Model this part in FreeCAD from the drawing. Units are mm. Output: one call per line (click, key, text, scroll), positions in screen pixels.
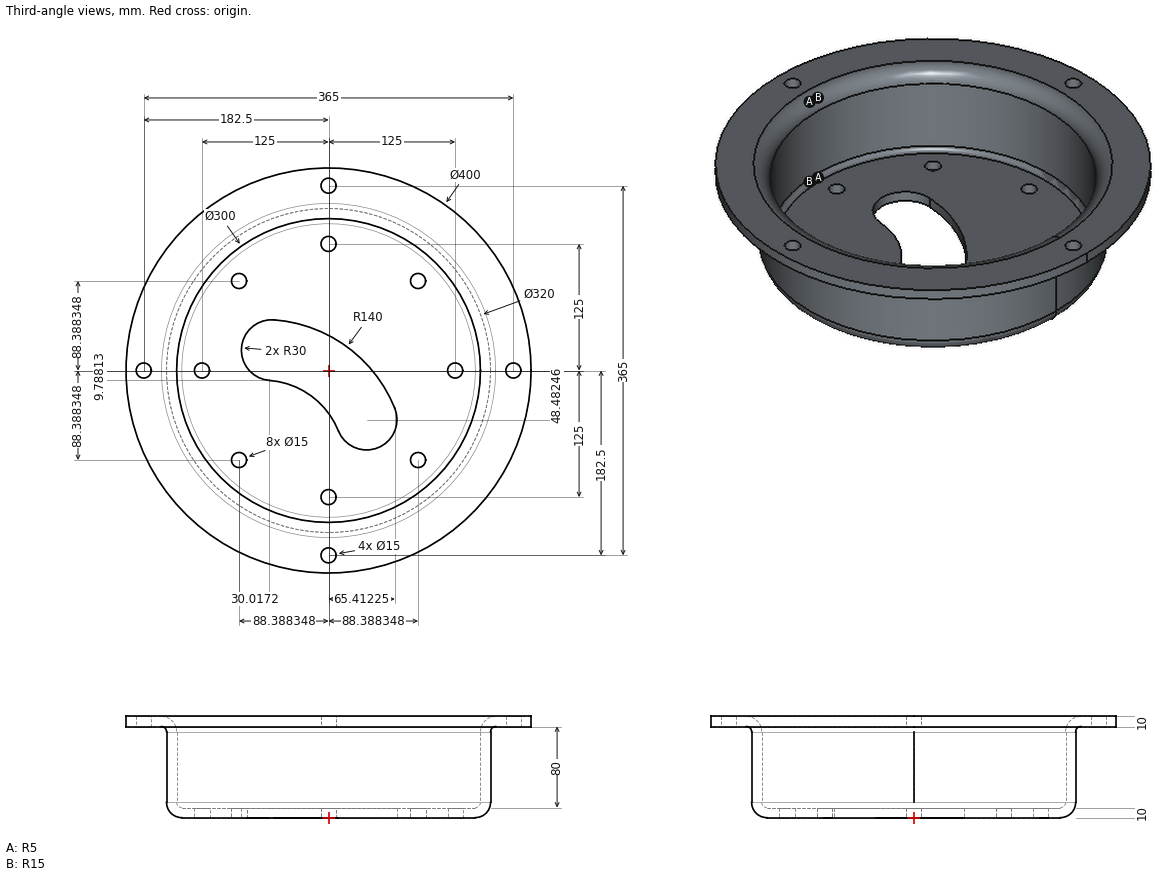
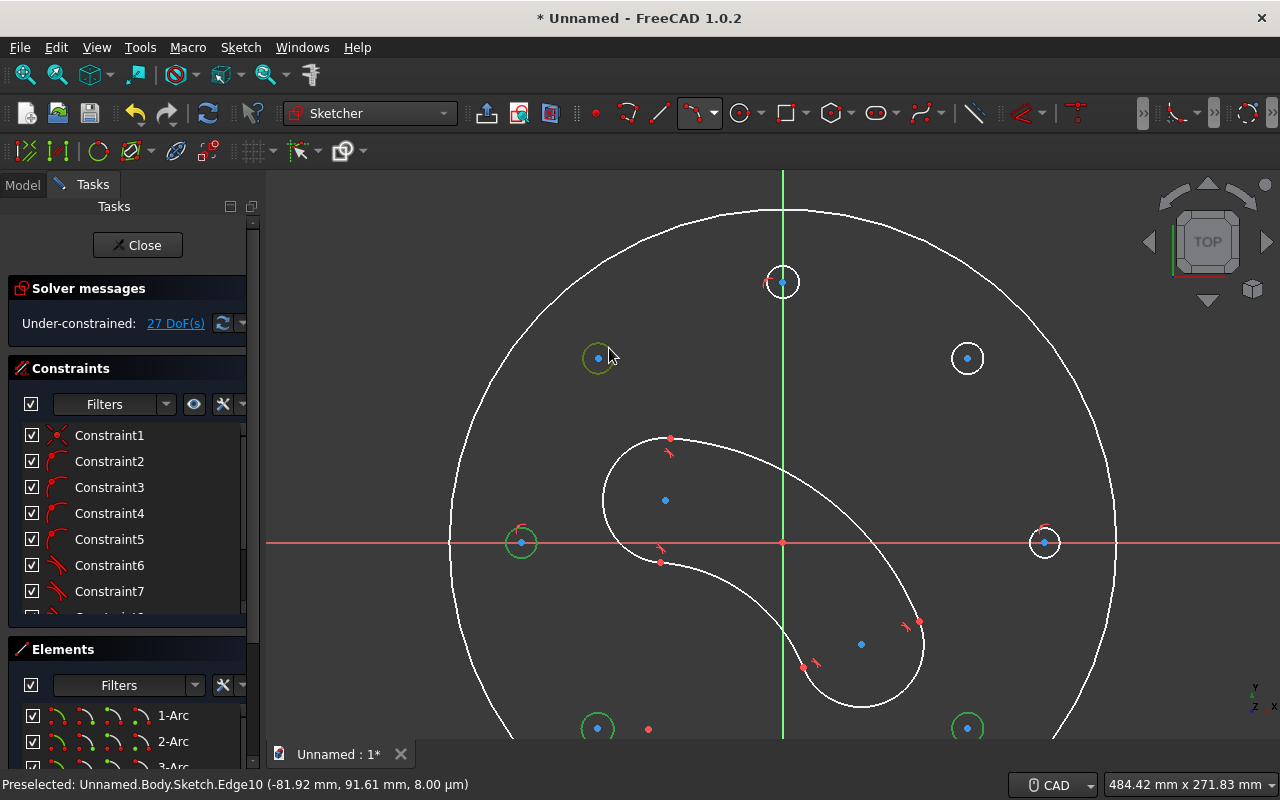
scroll(1055, 532, up, 2)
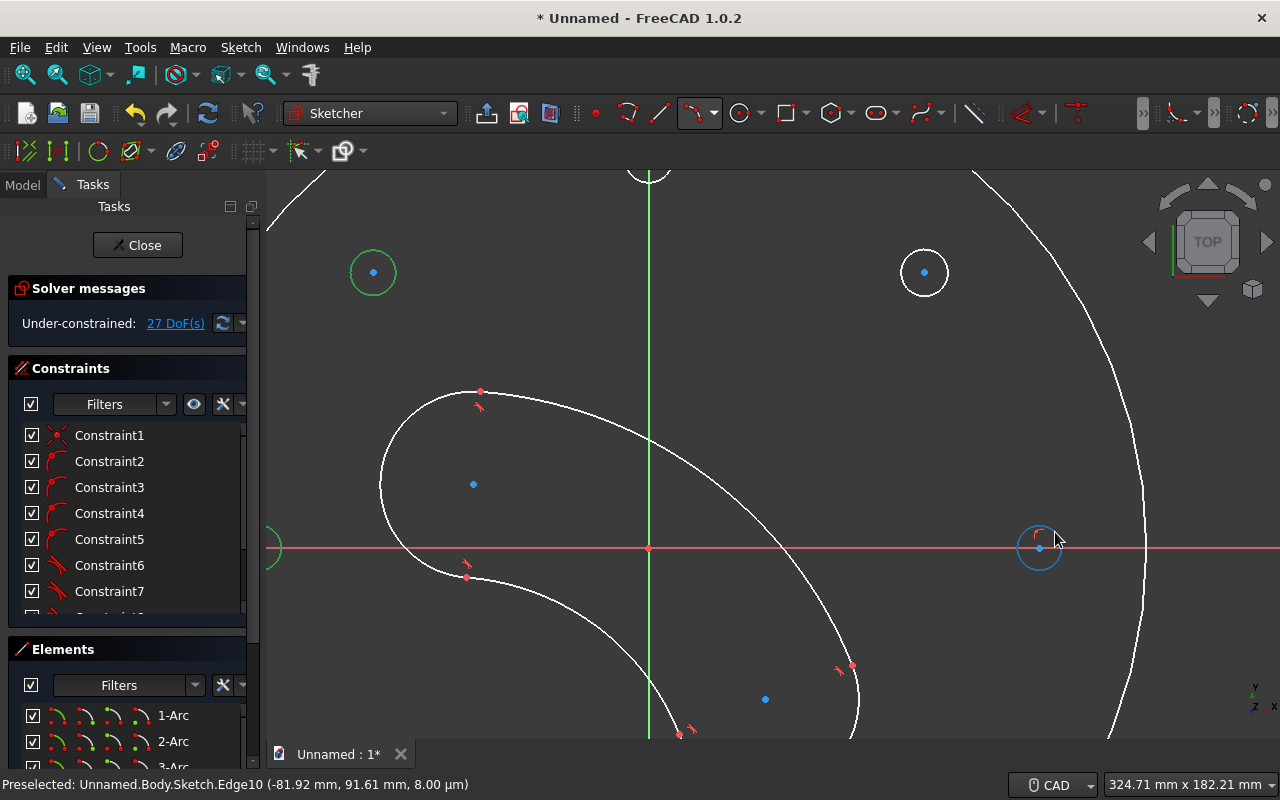
click(1055, 532)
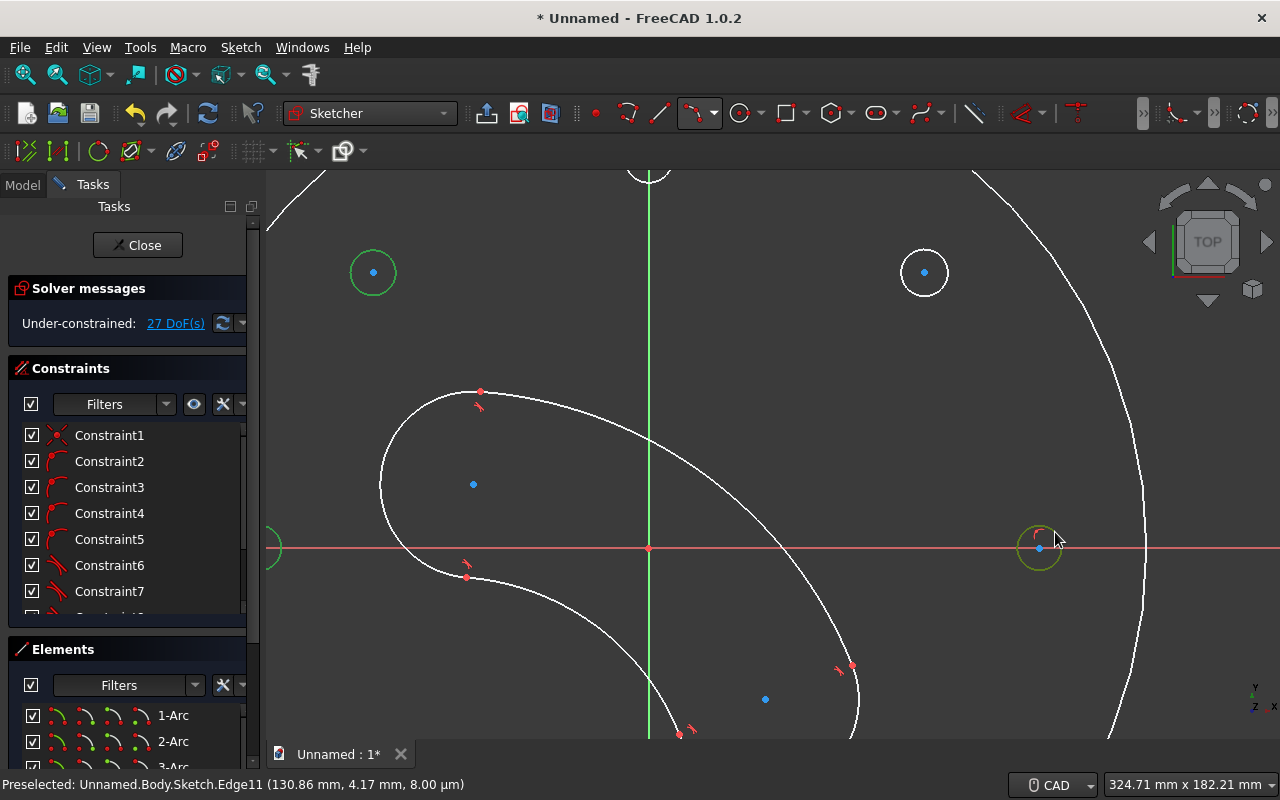
scroll(737, 400, down, 5)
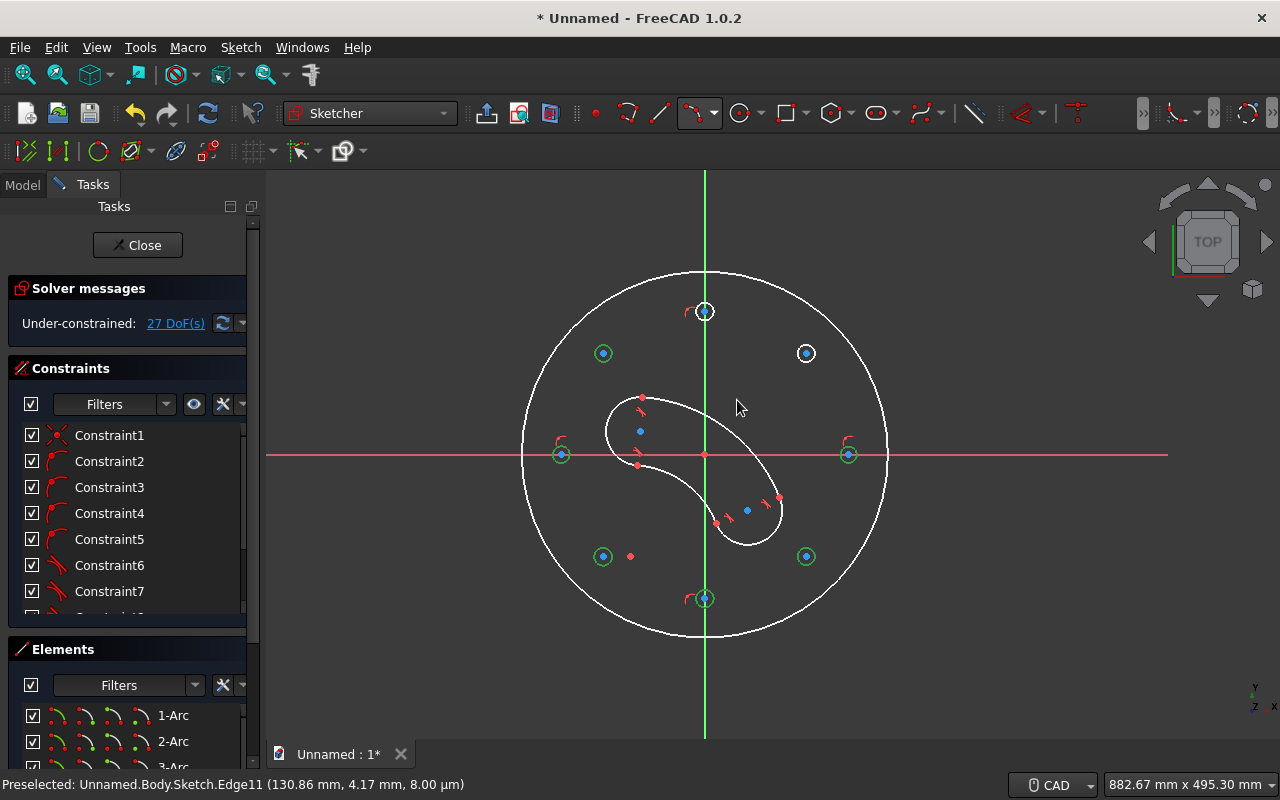
scroll(711, 305, up, 5)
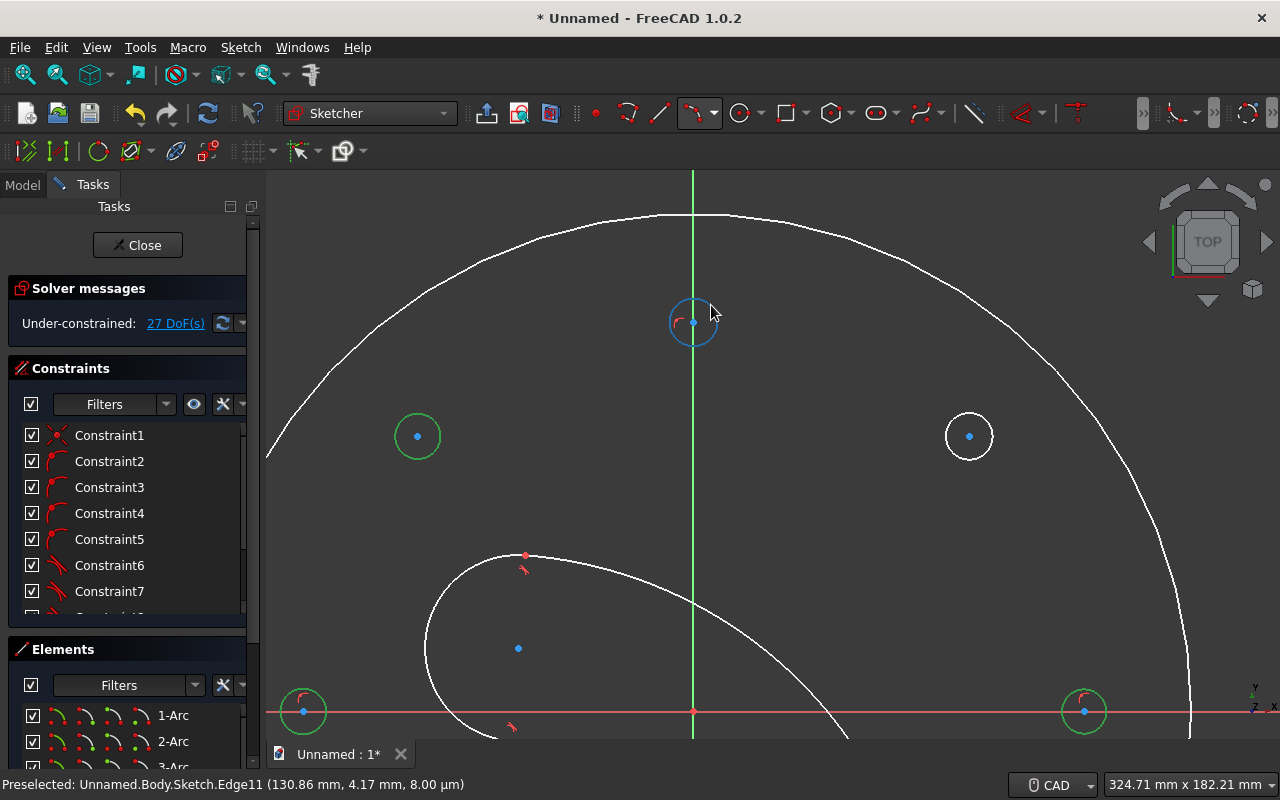
click(710, 305)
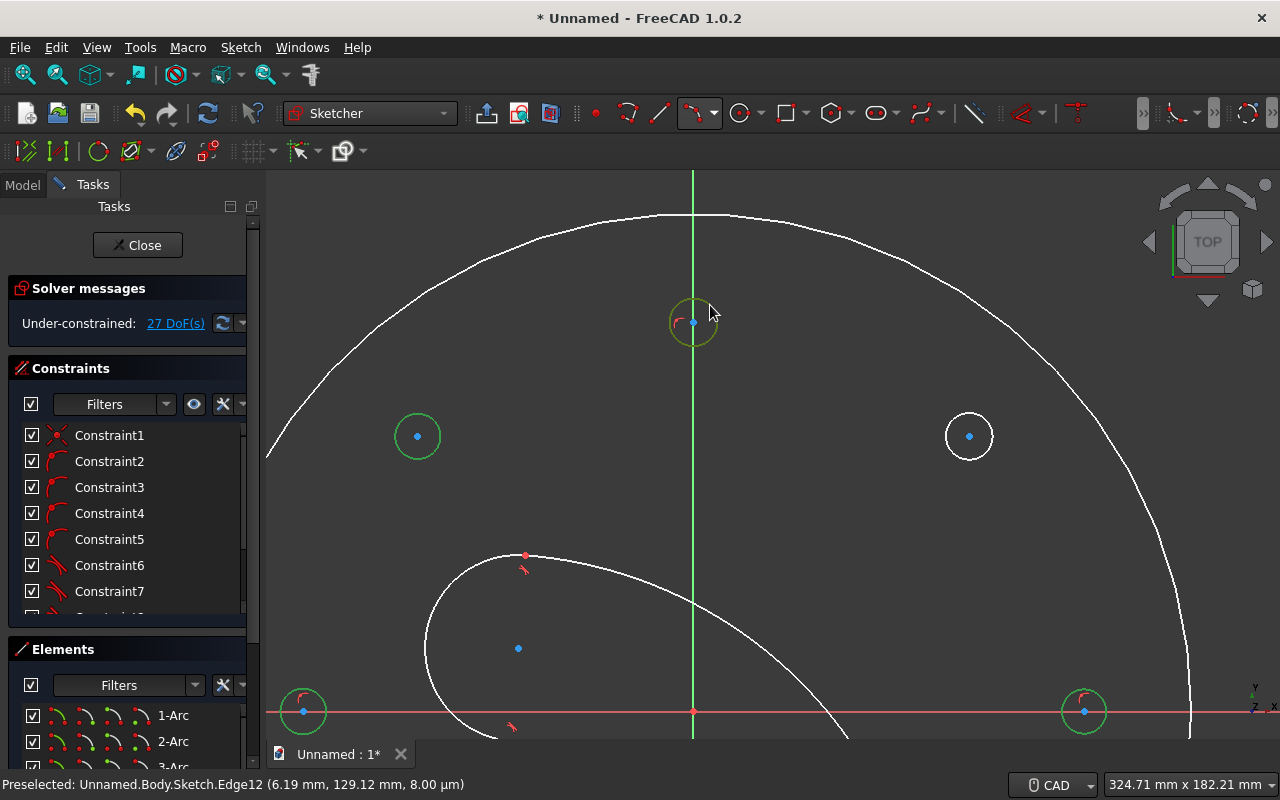
click(986, 420)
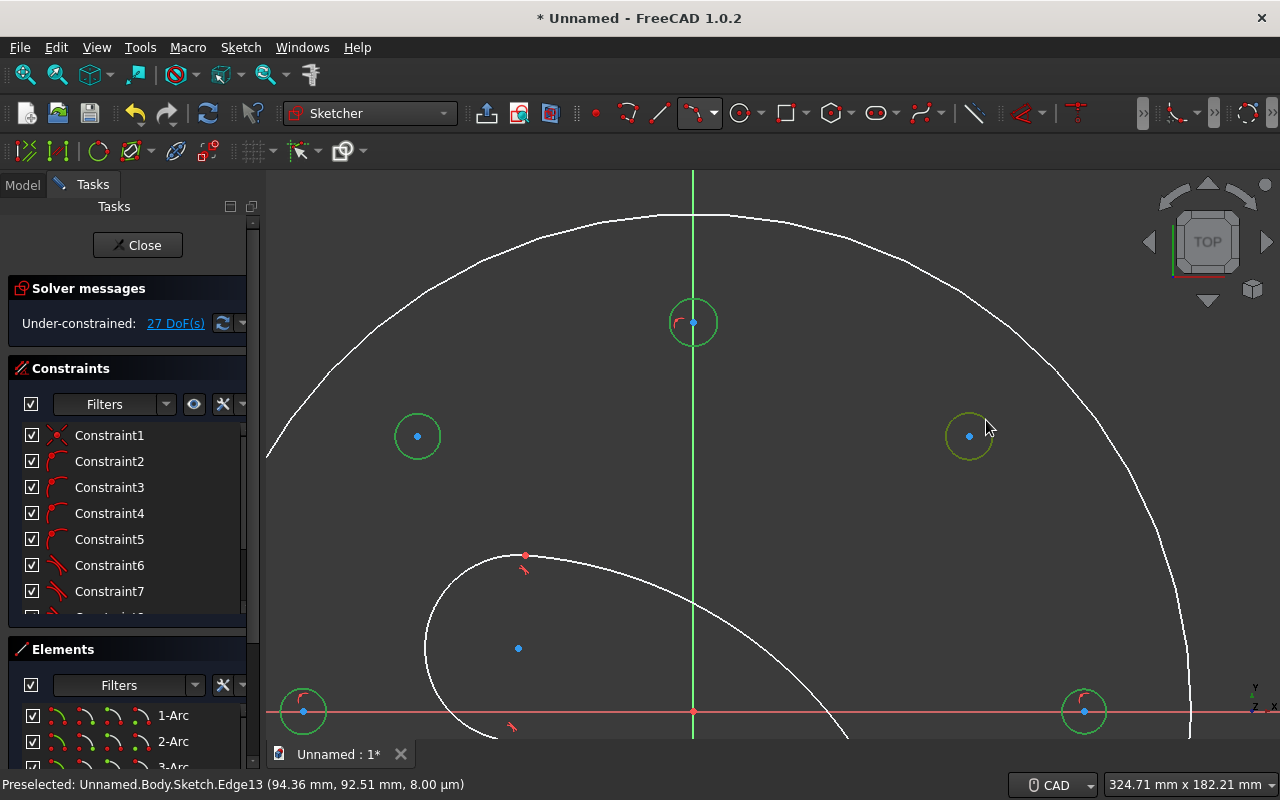
key(e)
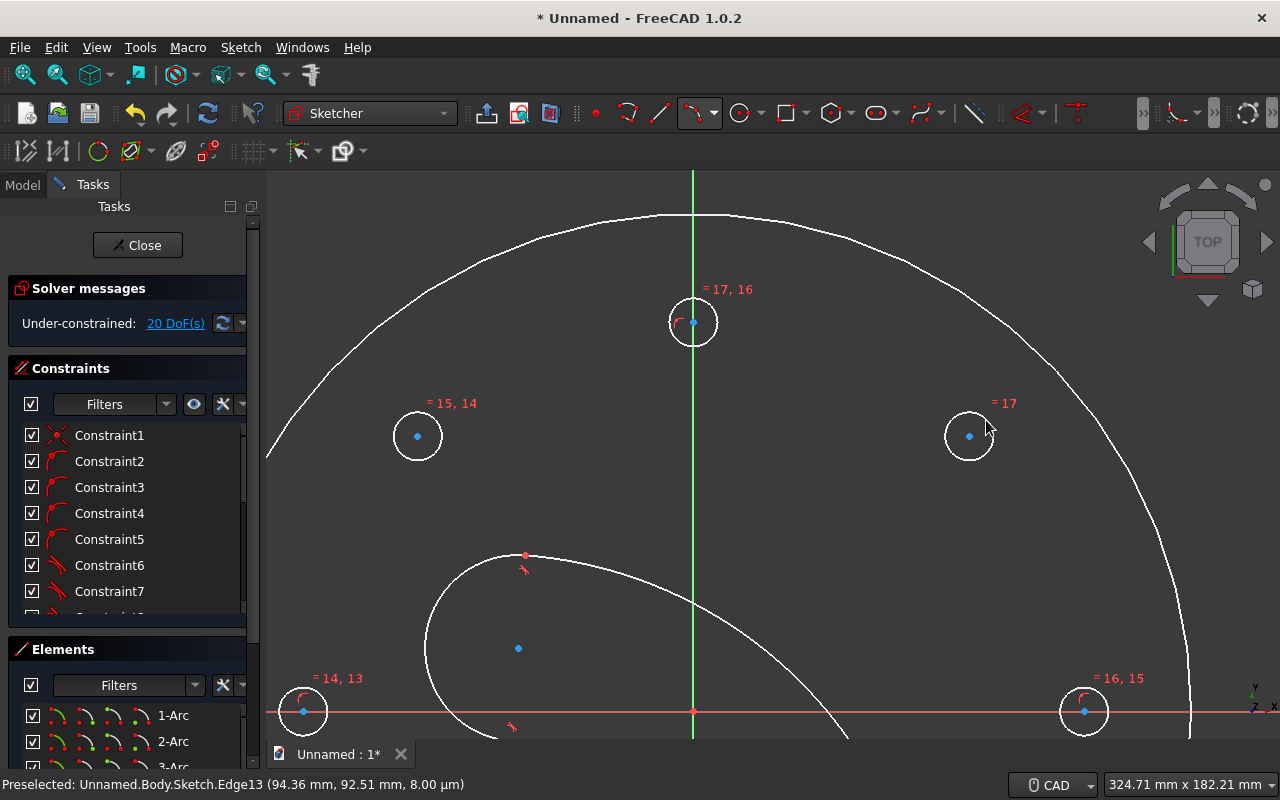
click(447, 588)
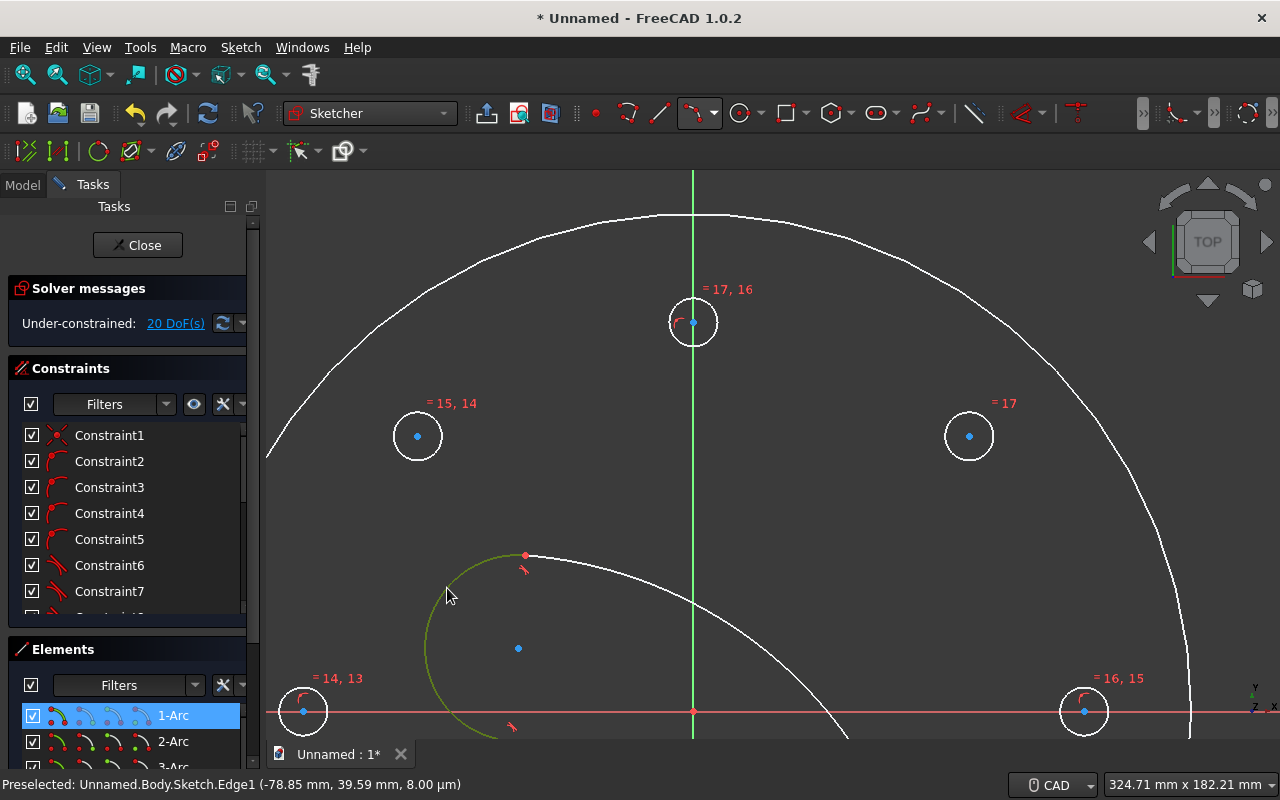
click(1044, 114)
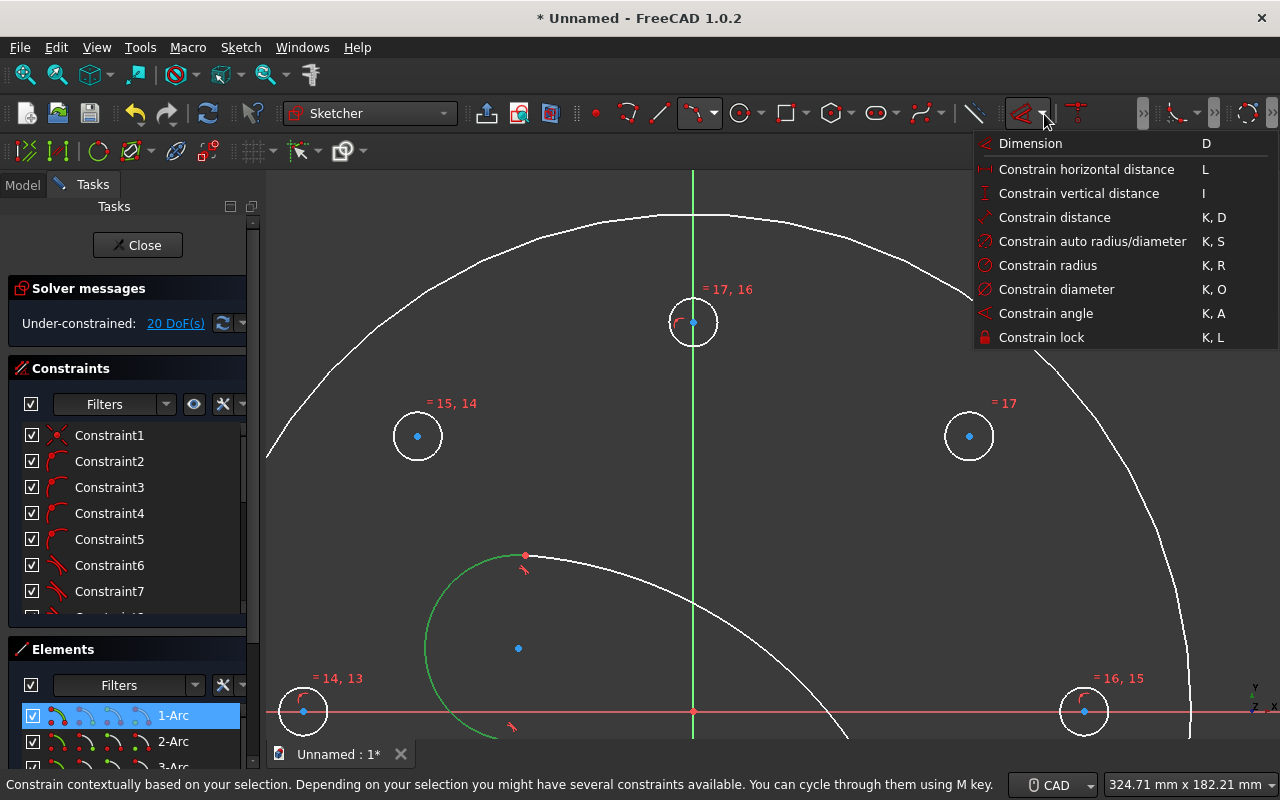
click(1126, 265)